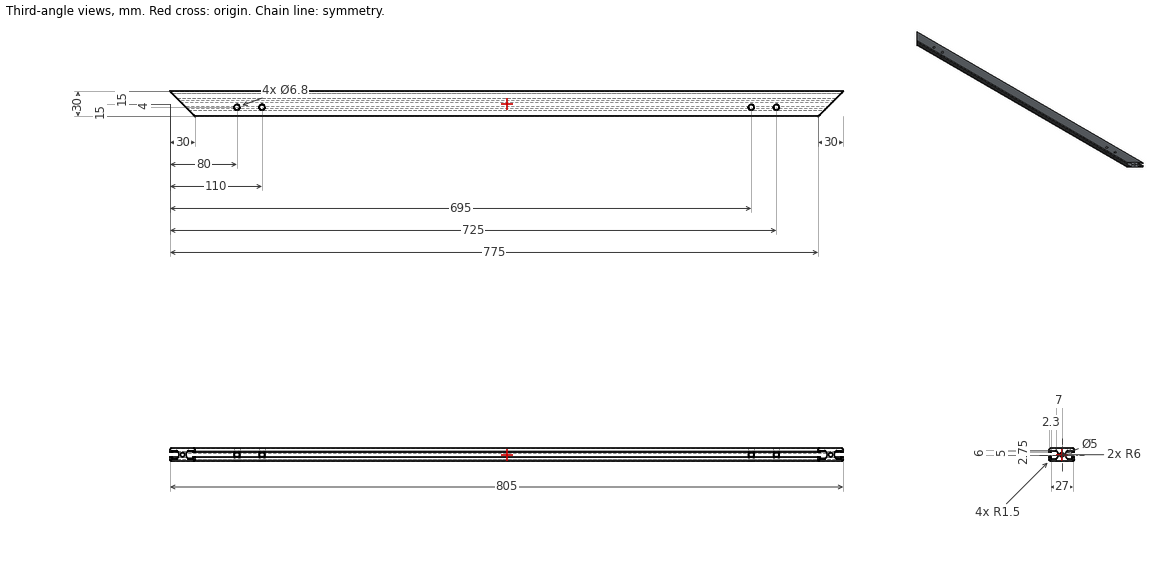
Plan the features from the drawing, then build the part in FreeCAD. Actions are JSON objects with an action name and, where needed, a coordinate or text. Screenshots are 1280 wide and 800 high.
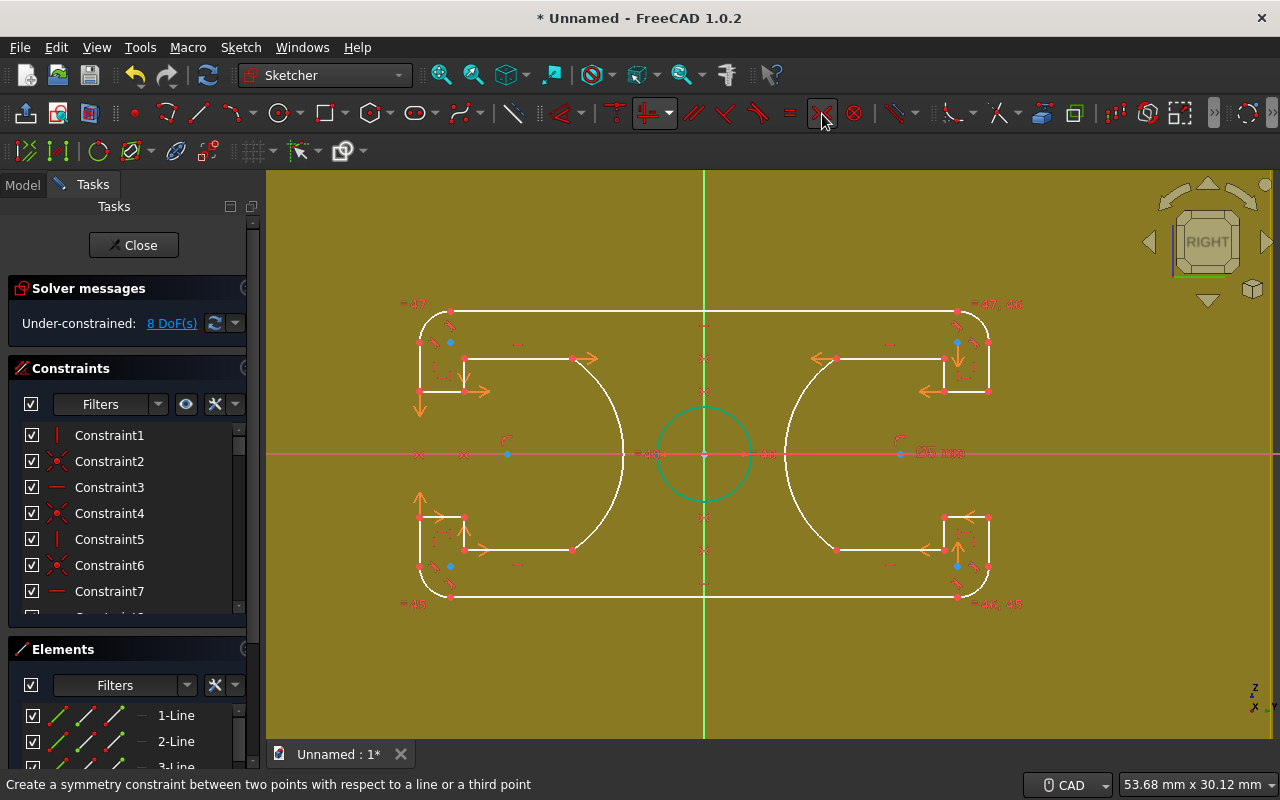
{"action": "left_click", "coordinate": [615, 498]}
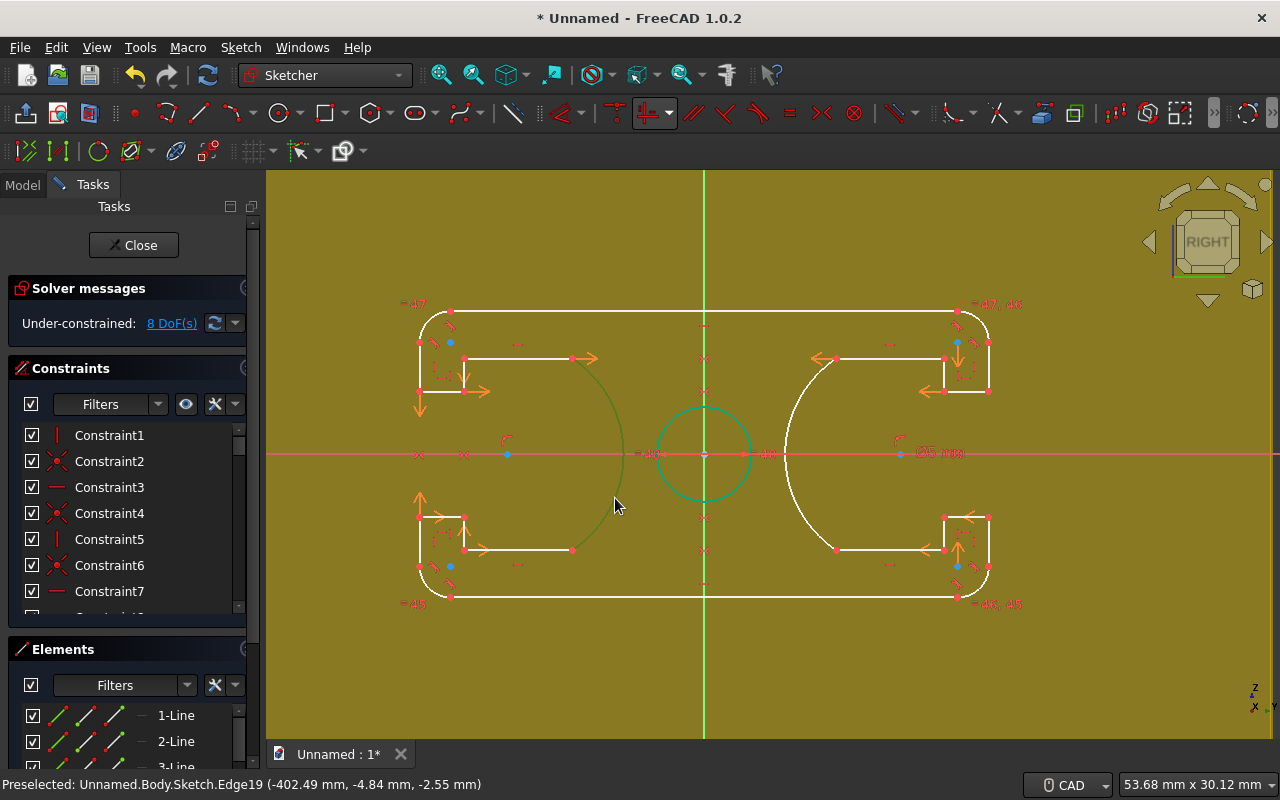
{"action": "key", "text": "k r"}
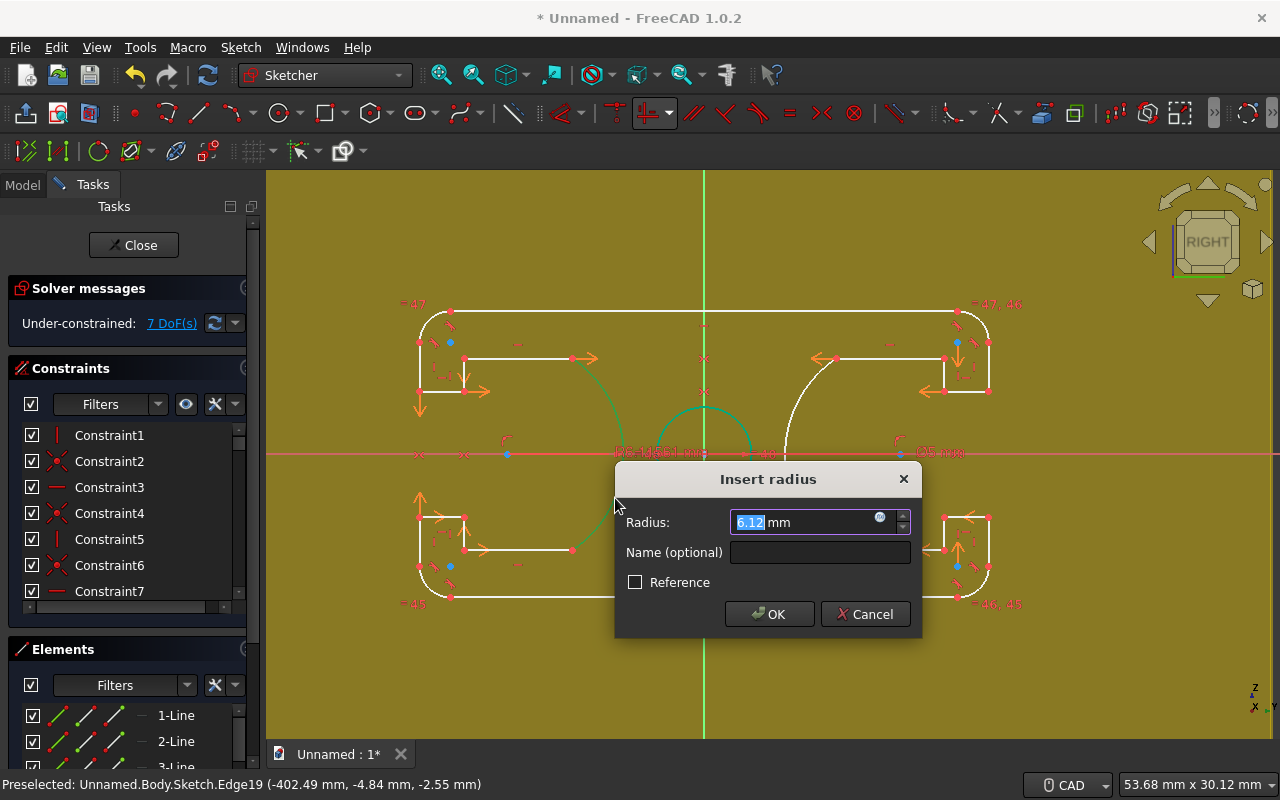
{"action": "type", "text": "6"}
{"action": "key", "text": "Return"}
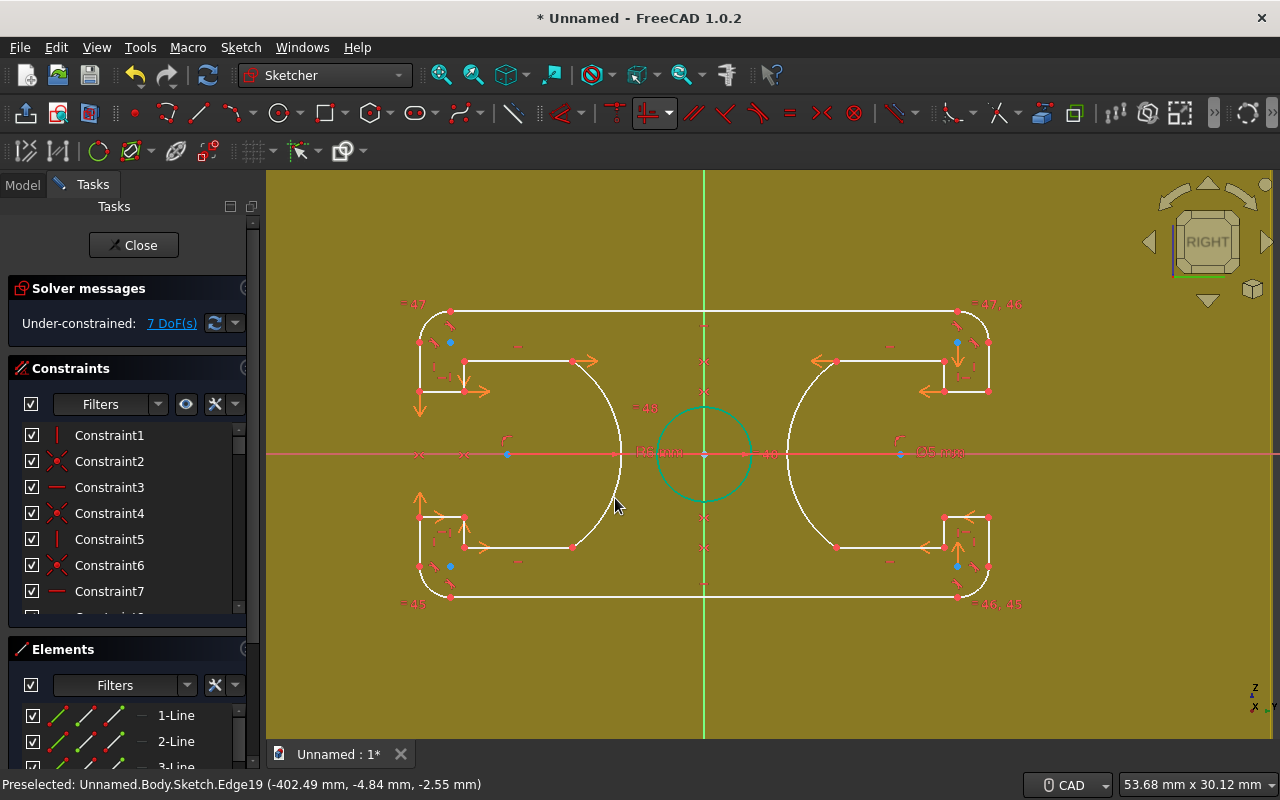
{"action": "scroll", "coordinate": [423, 581], "scroll_direction": "up", "scroll_amount": 2}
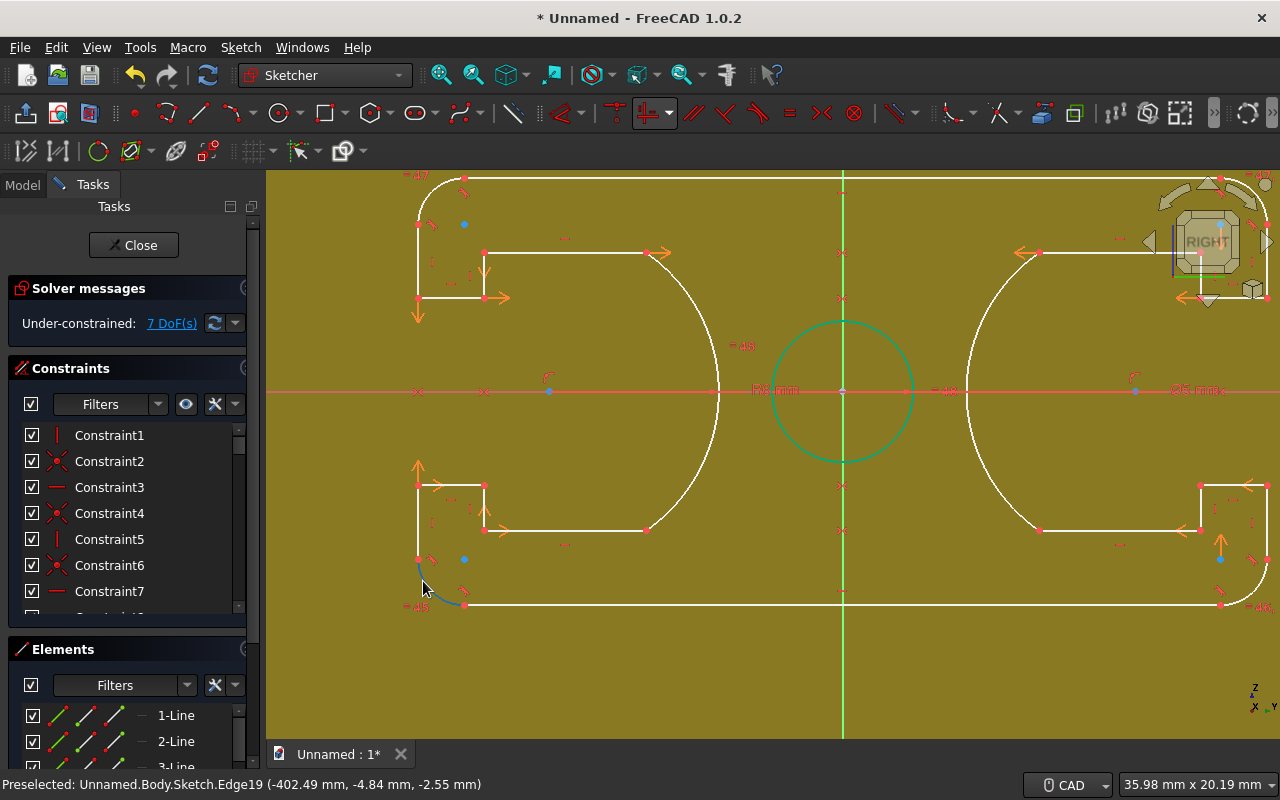
{"action": "left_click", "coordinate": [423, 580]}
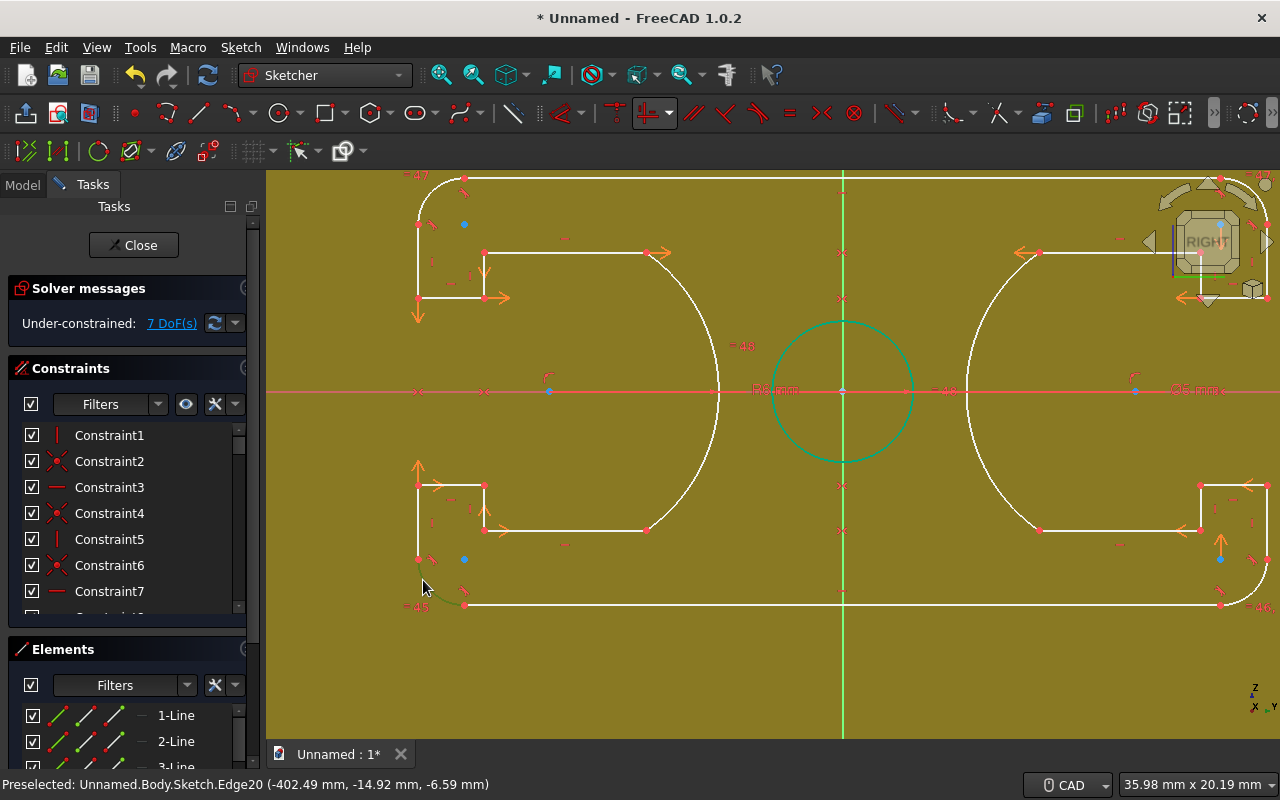
{"action": "left_click", "coordinate": [584, 114]}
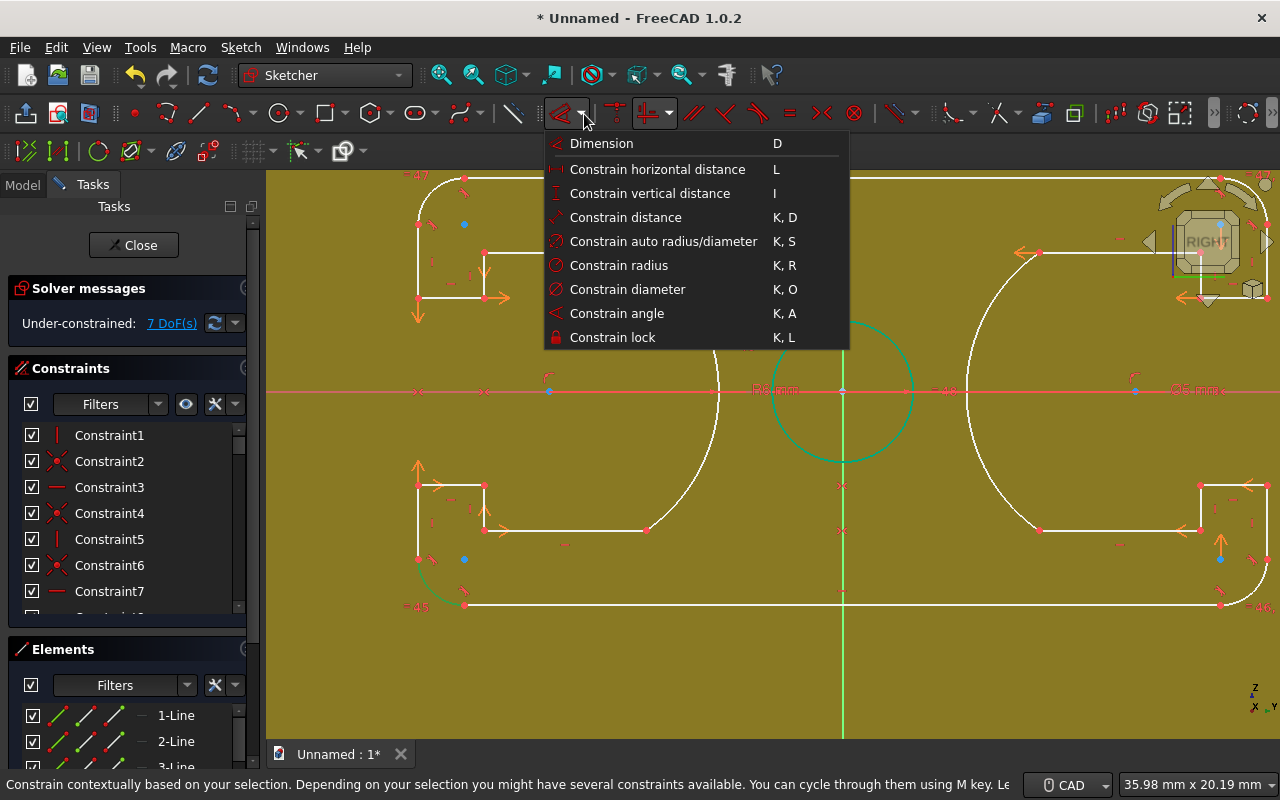
{"action": "left_click", "coordinate": [697, 265]}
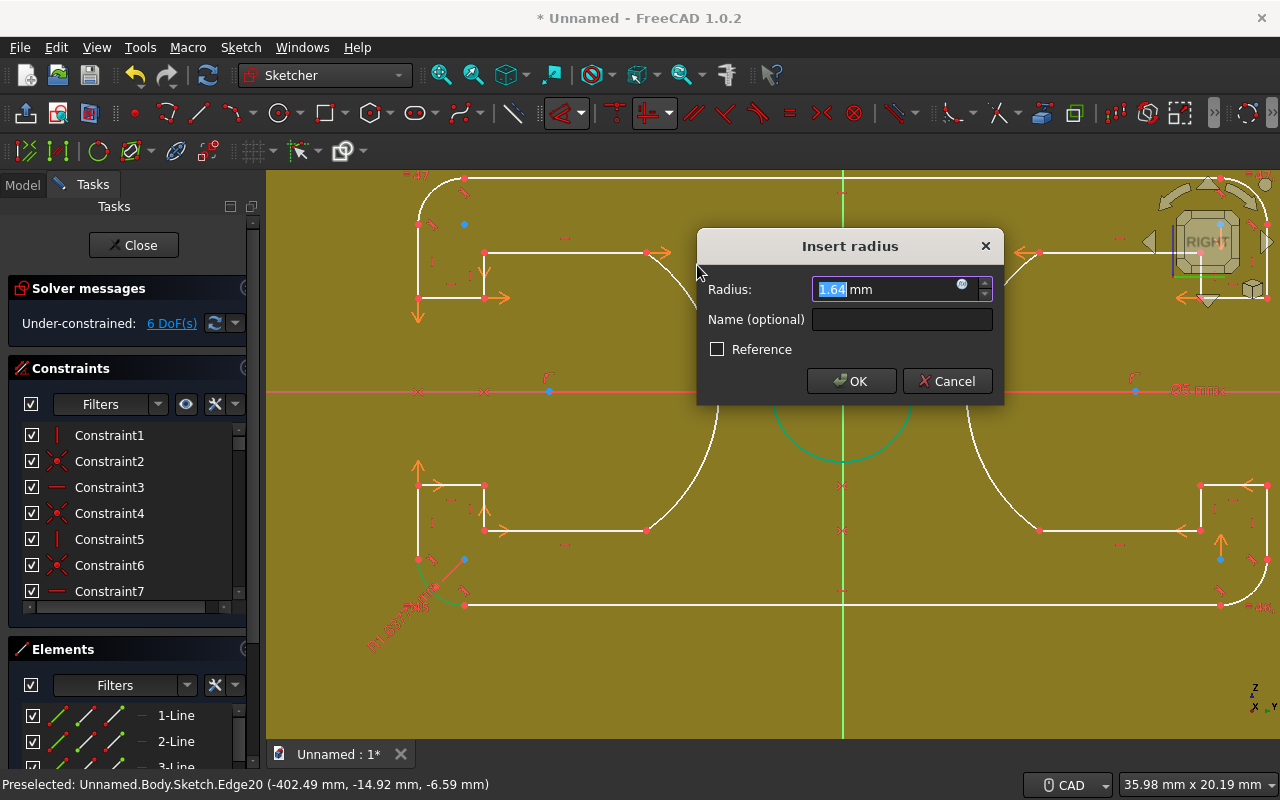
{"action": "type", "text": "1.5"}
{"action": "key", "text": "Return"}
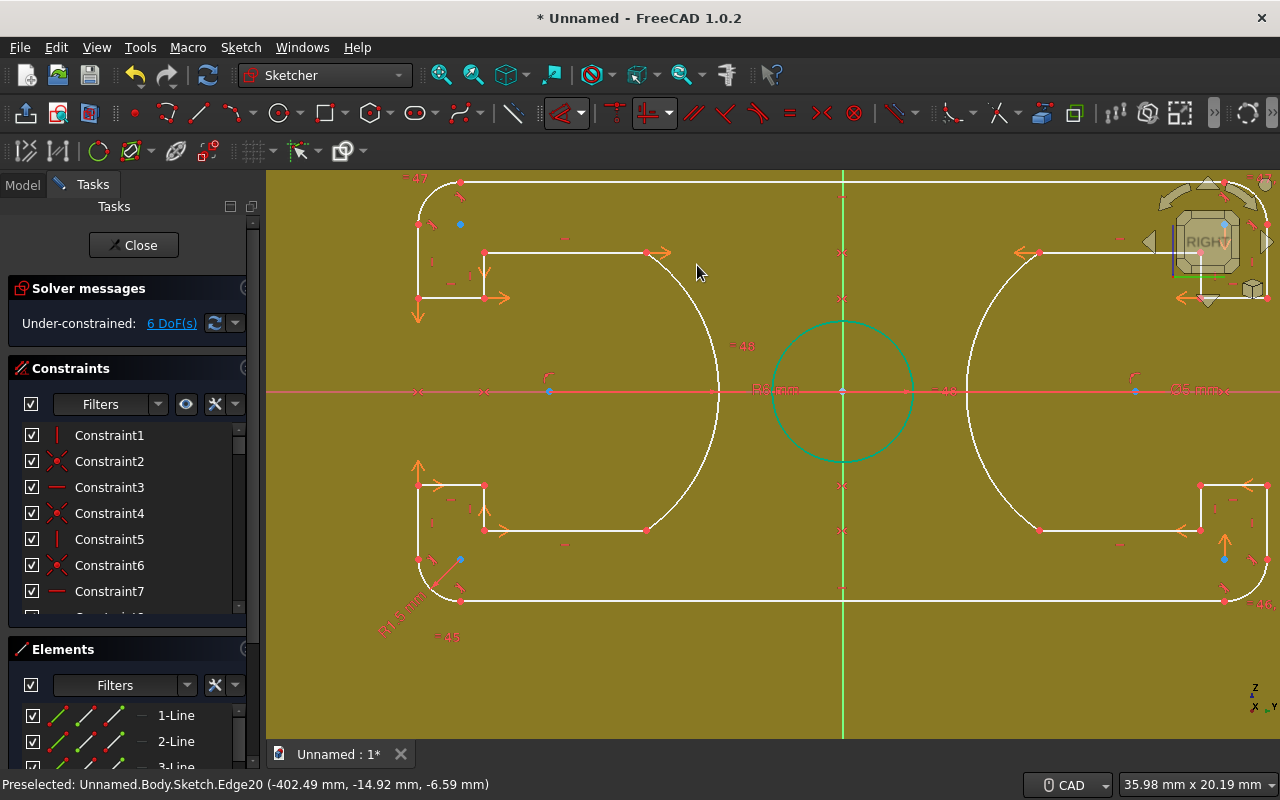
{"action": "left_click", "coordinate": [690, 601]}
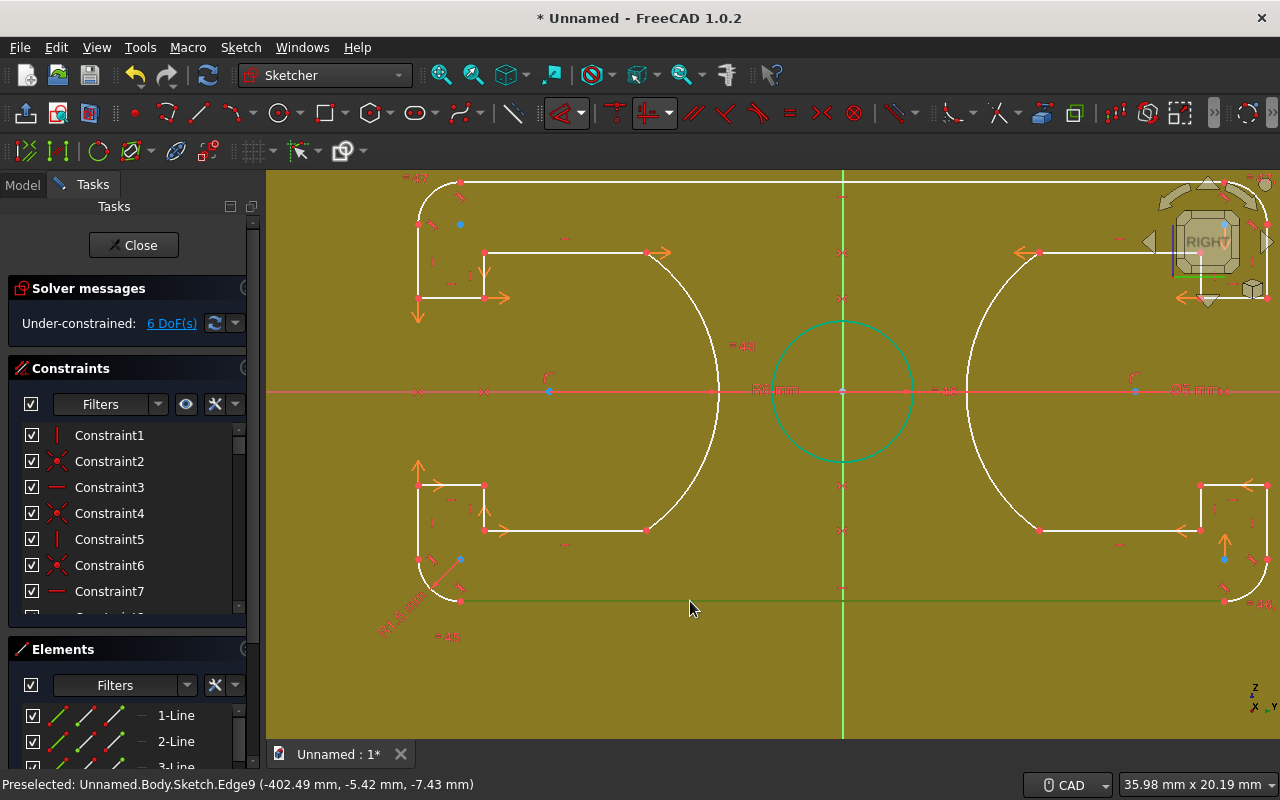
{"action": "left_click", "coordinate": [584, 114]}